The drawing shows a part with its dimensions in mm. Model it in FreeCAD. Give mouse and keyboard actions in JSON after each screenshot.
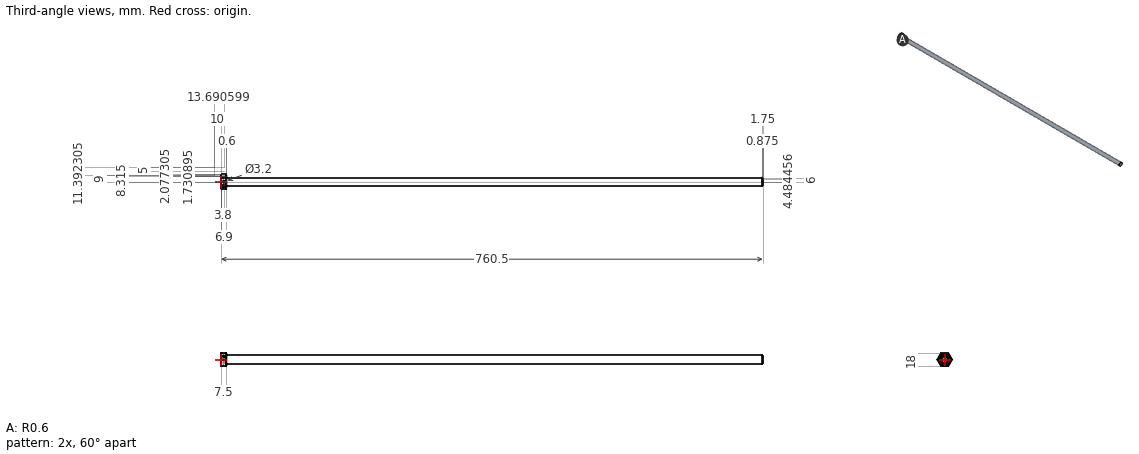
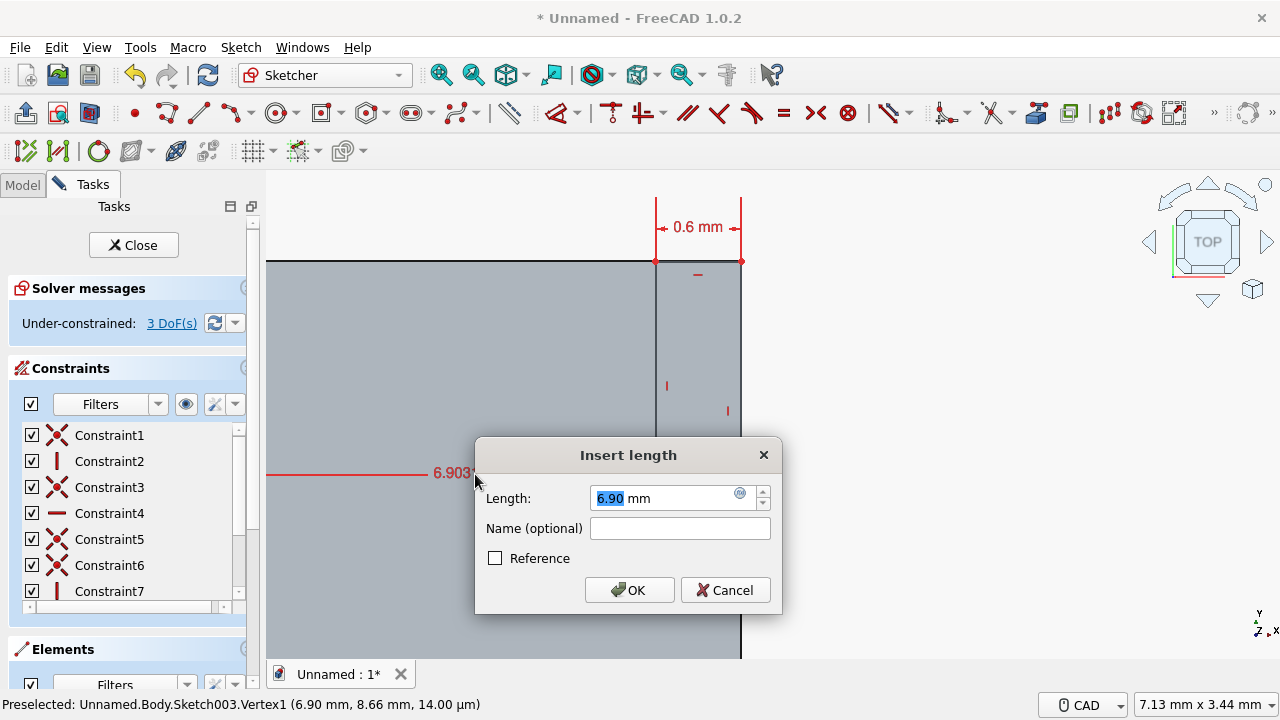
{"action": "type", "text": "6.9"}
{"action": "key", "text": "Return"}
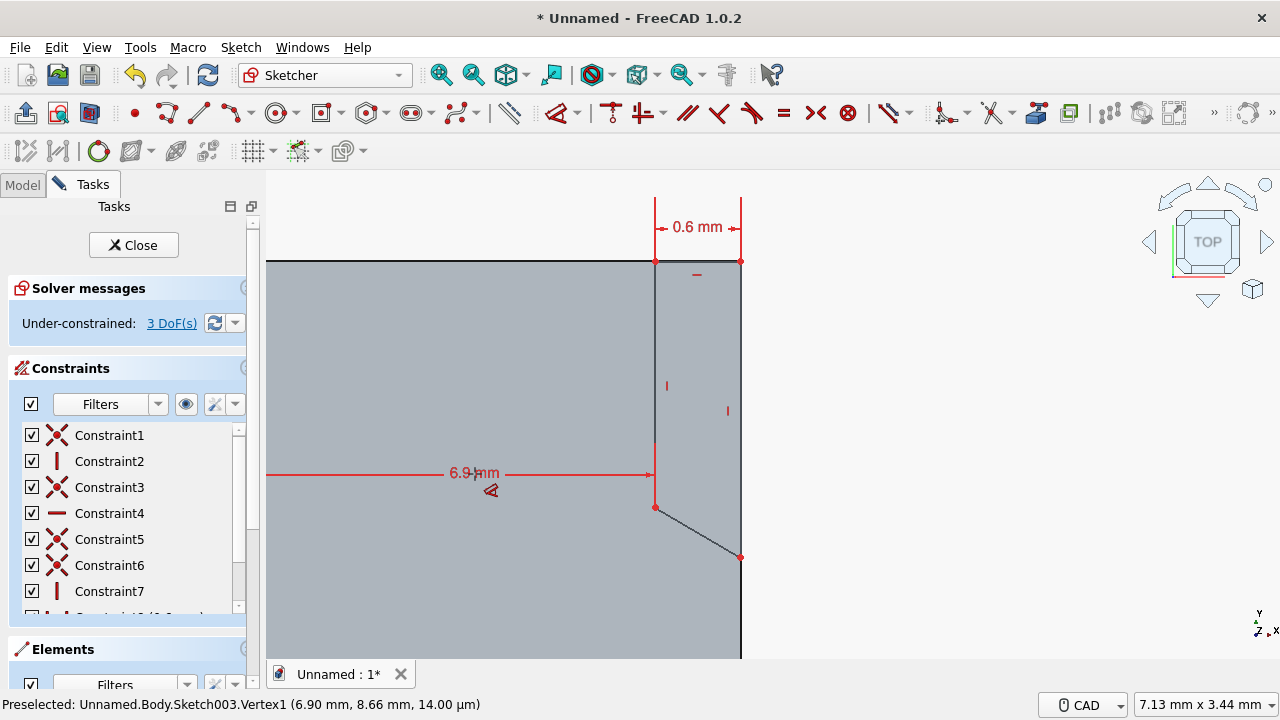
{"action": "left_click", "coordinate": [741, 558]}
{"action": "left_click", "coordinate": [775, 594]}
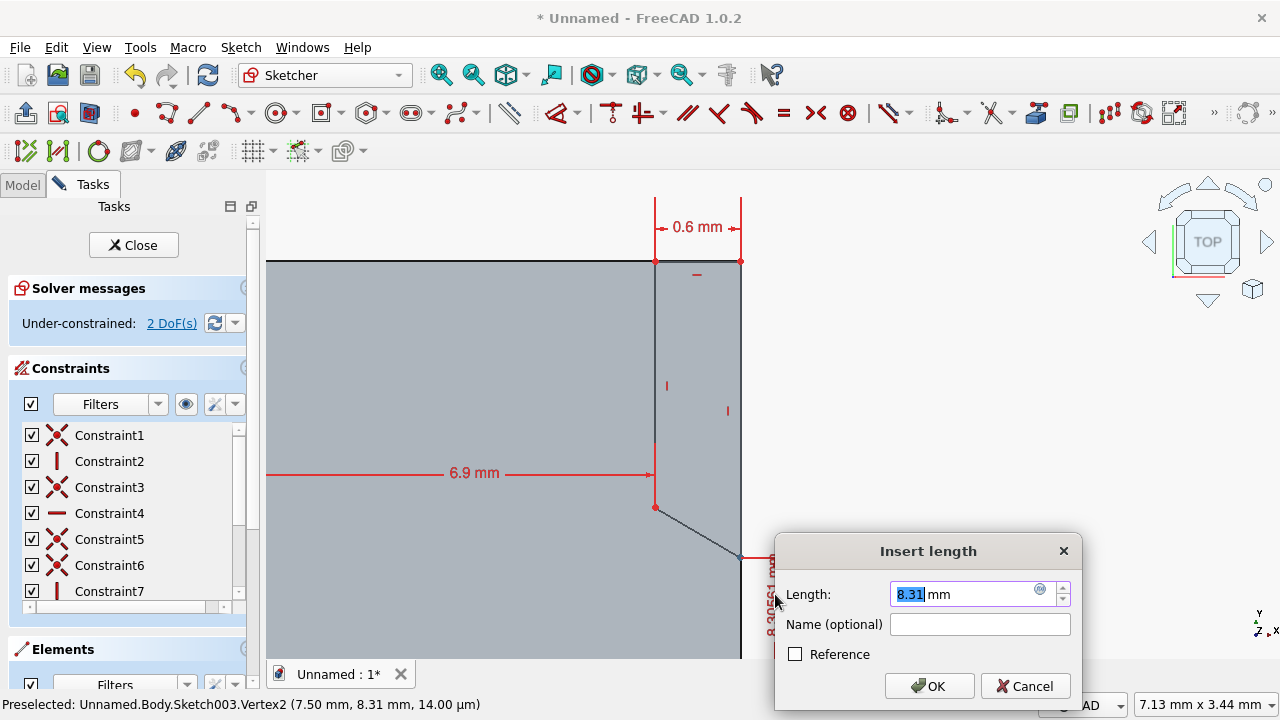
{"action": "type", "text": "8.315"}
{"action": "key", "text": "Return"}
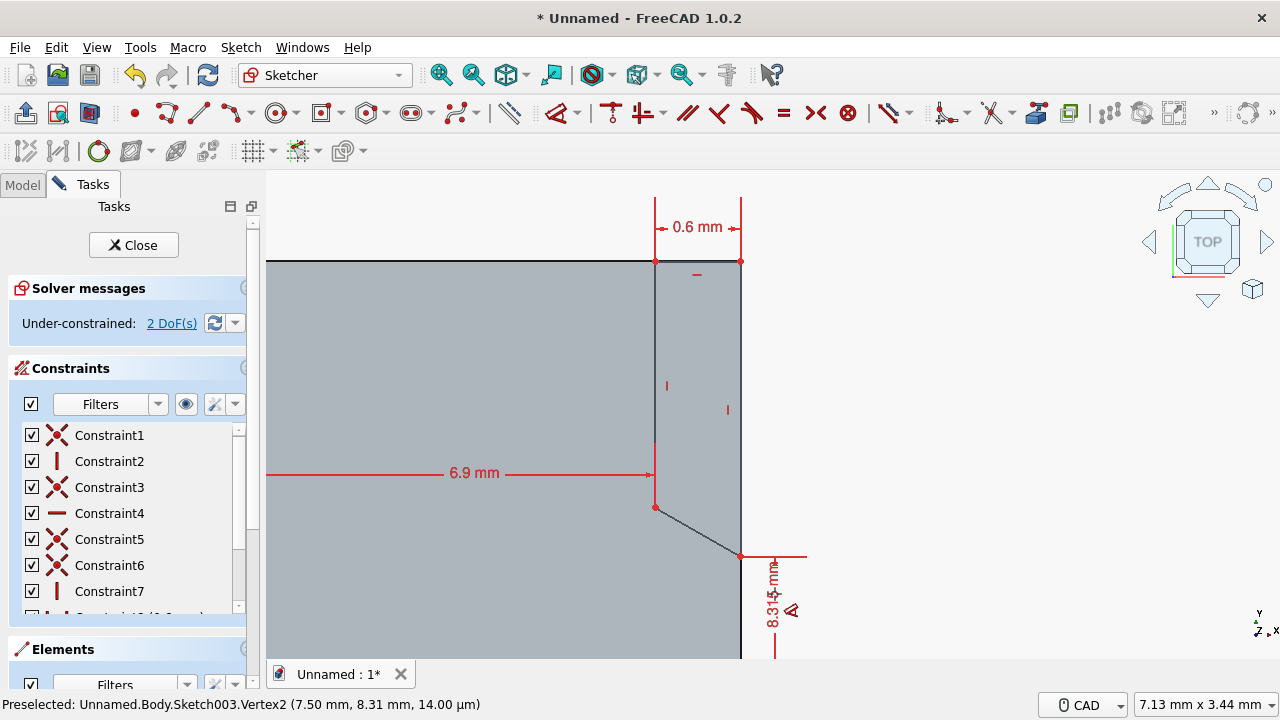
{"action": "left_click", "coordinate": [741, 468]}
{"action": "left_click", "coordinate": [775, 409]}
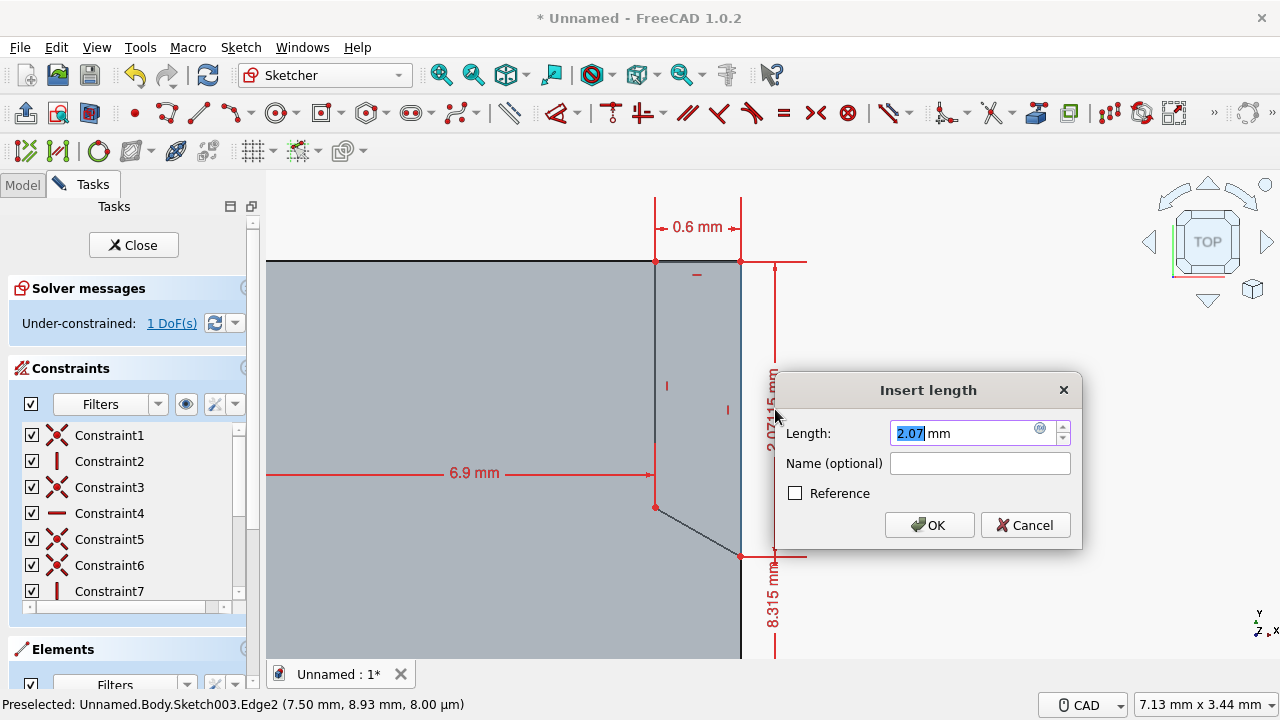
{"action": "type", "text": "2.077305"}
{"action": "key", "text": "Return"}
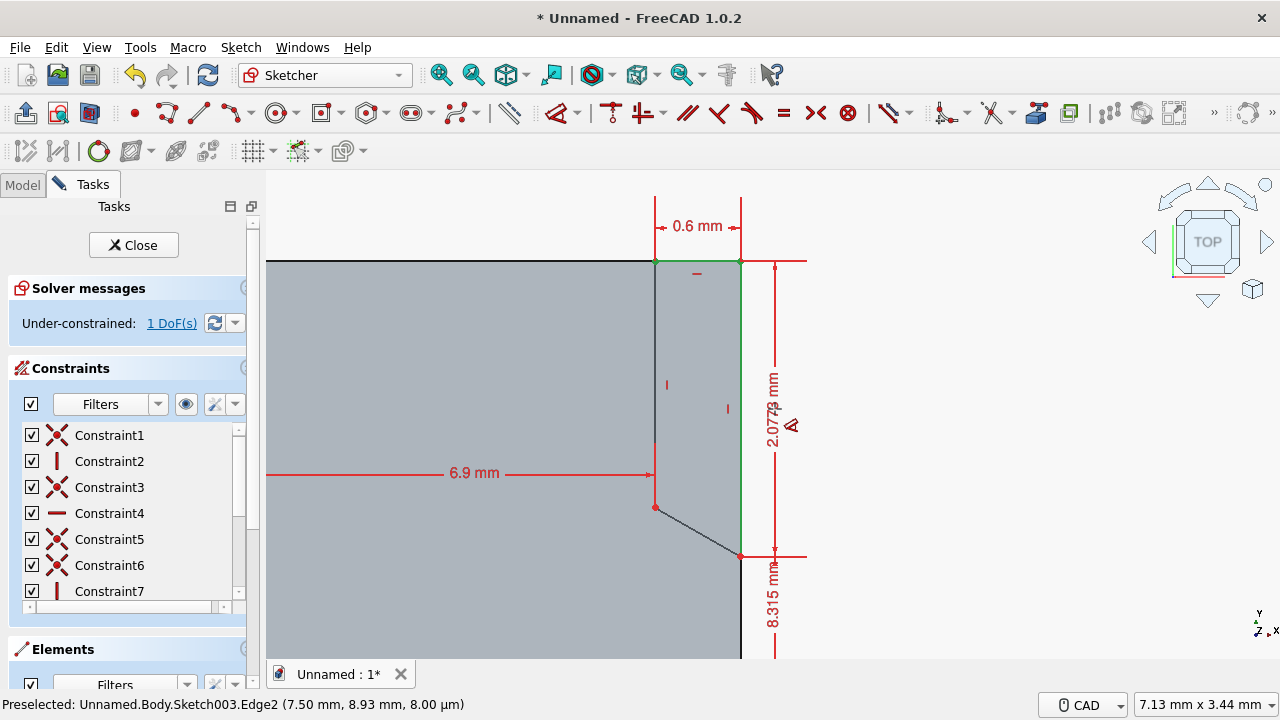
{"action": "left_click", "coordinate": [655, 335]}
{"action": "left_click", "coordinate": [621, 385]}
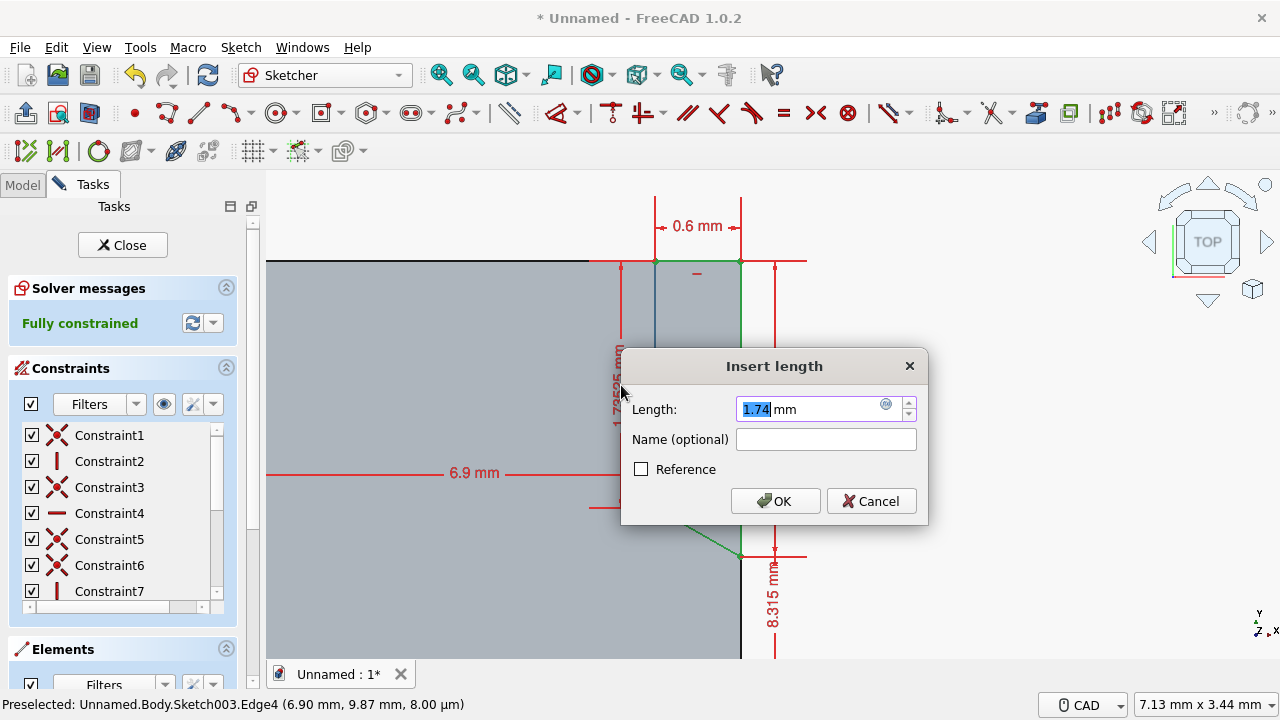
{"action": "type", "text": "1.730895"}
{"action": "key", "text": "Return"}
{"action": "key", "text": "Escape"}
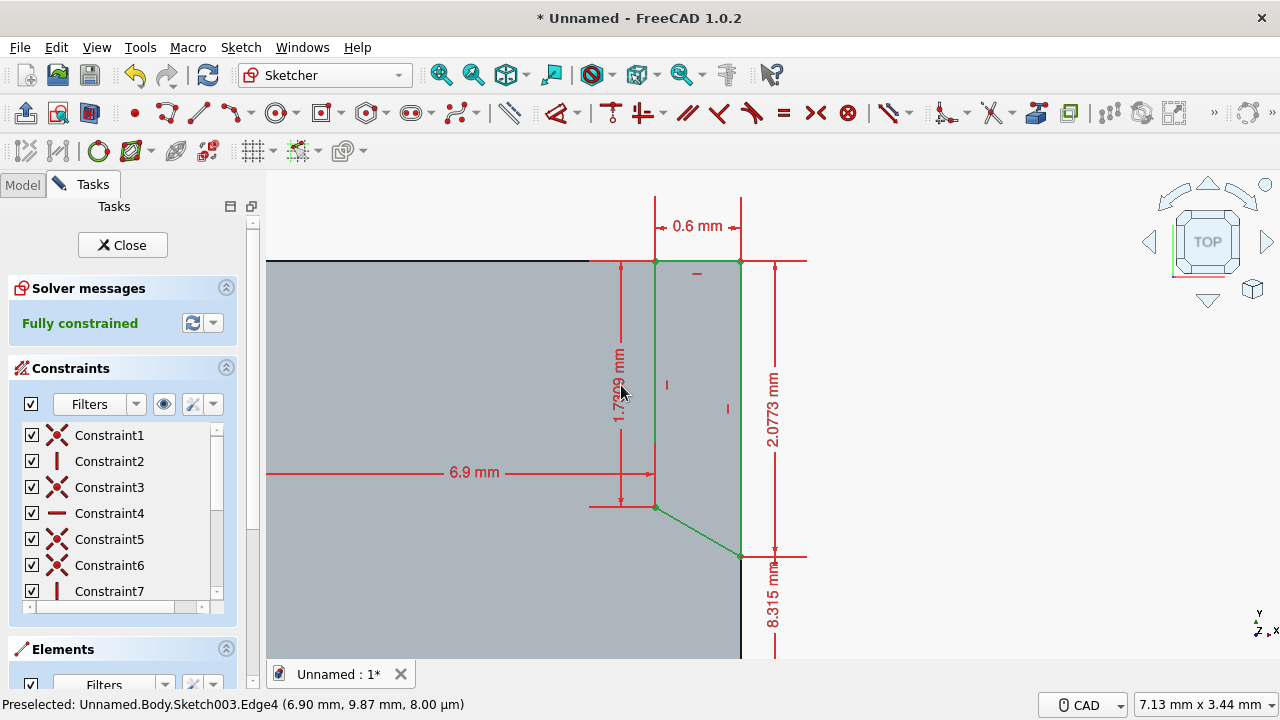
{"action": "left_click", "coordinate": [123, 245]}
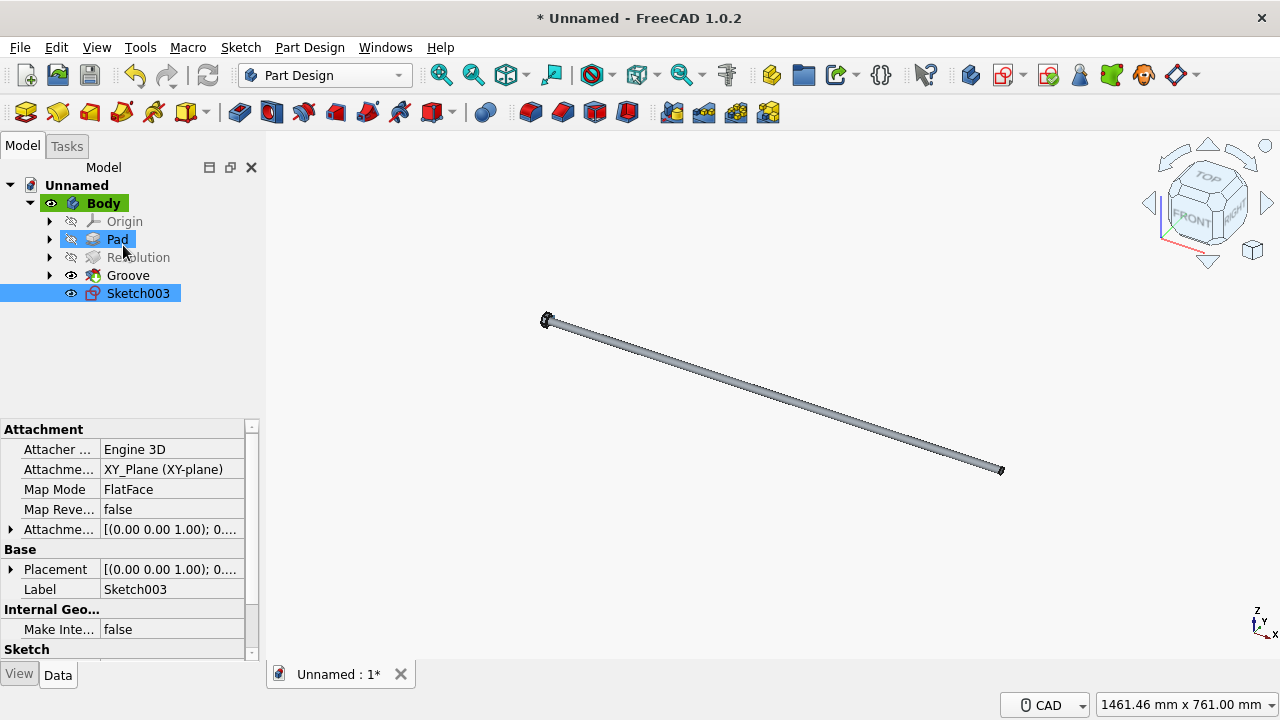
{"action": "left_click", "coordinate": [304, 112]}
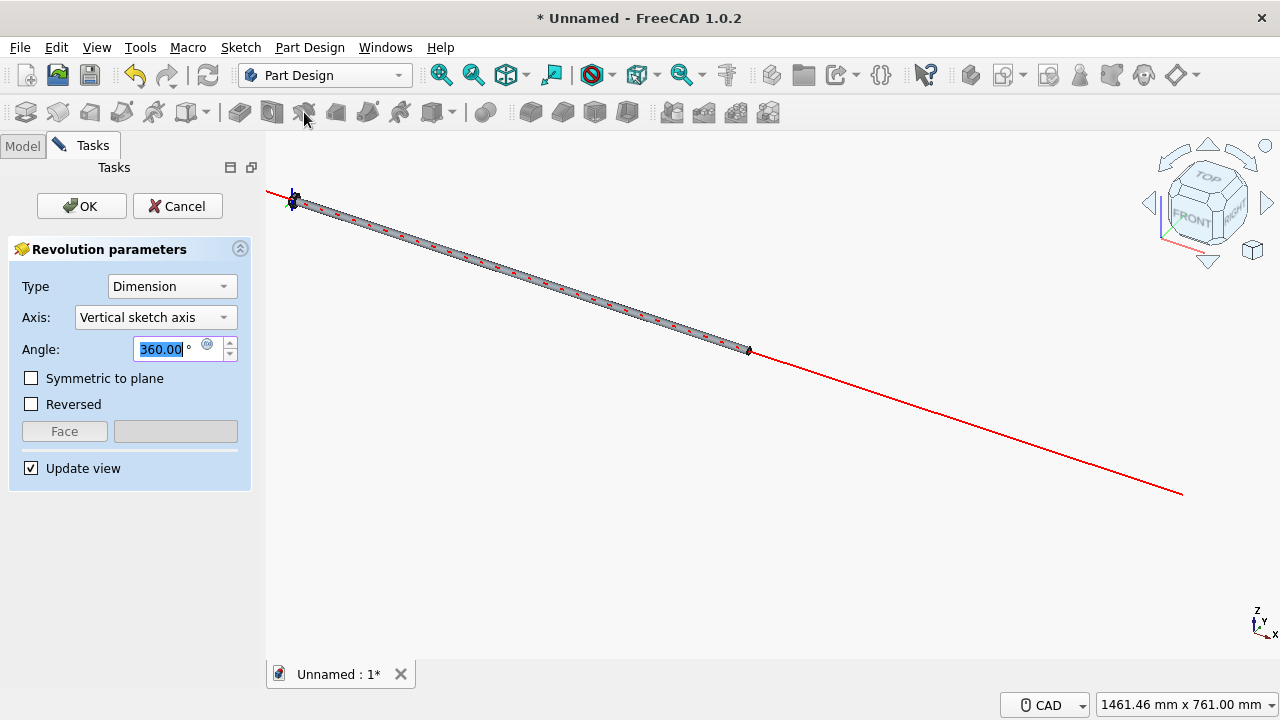
{"action": "left_click", "coordinate": [156, 318]}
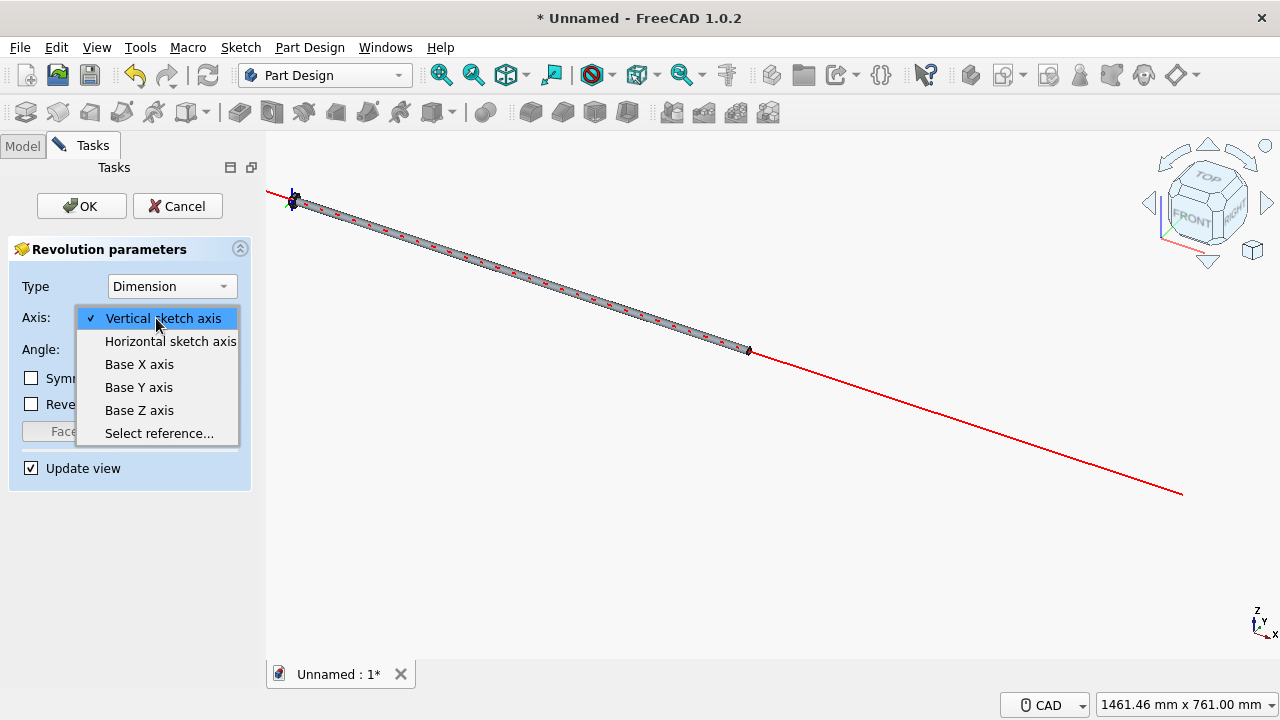
{"action": "left_click", "coordinate": [156, 342]}